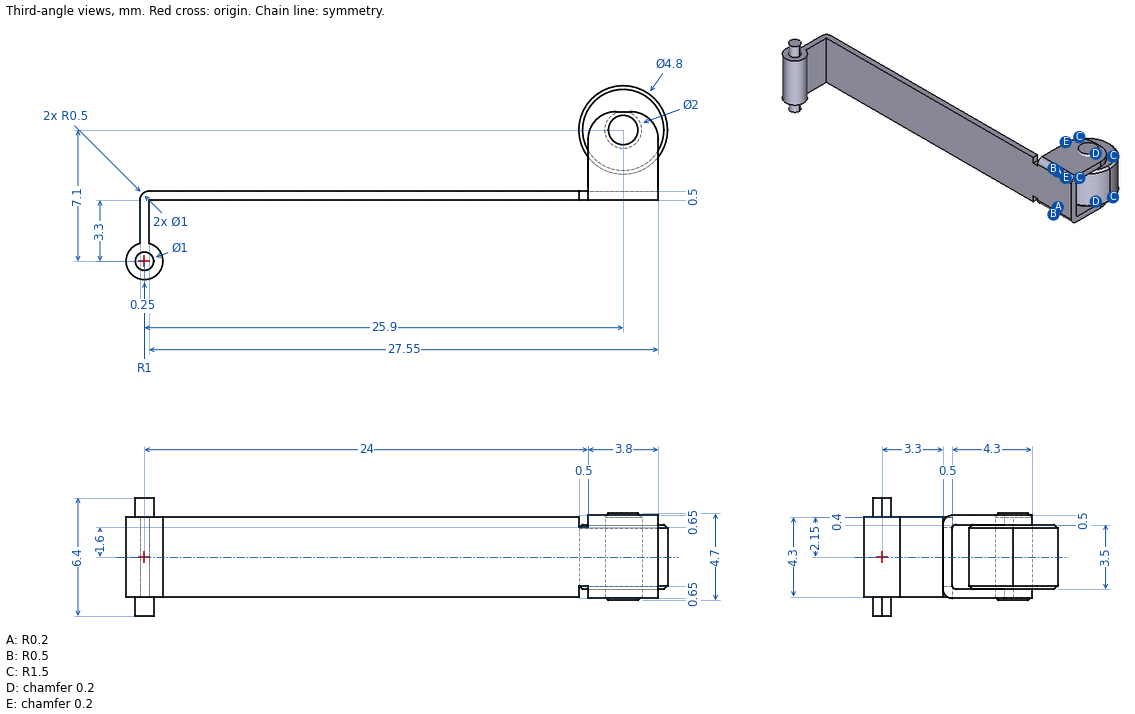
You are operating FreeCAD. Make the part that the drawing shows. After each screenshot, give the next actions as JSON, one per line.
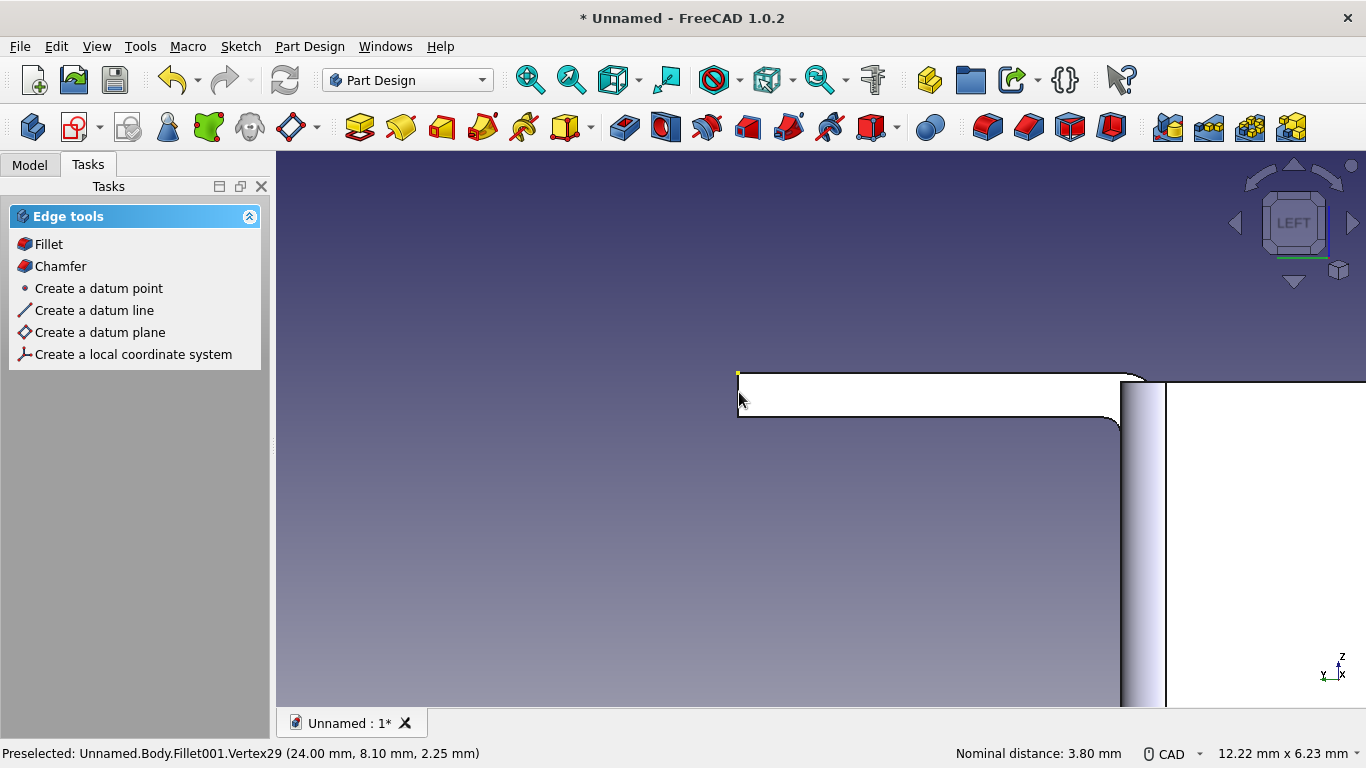
{"action": "left_click", "coordinate": [738, 394], "text": "ctrl"}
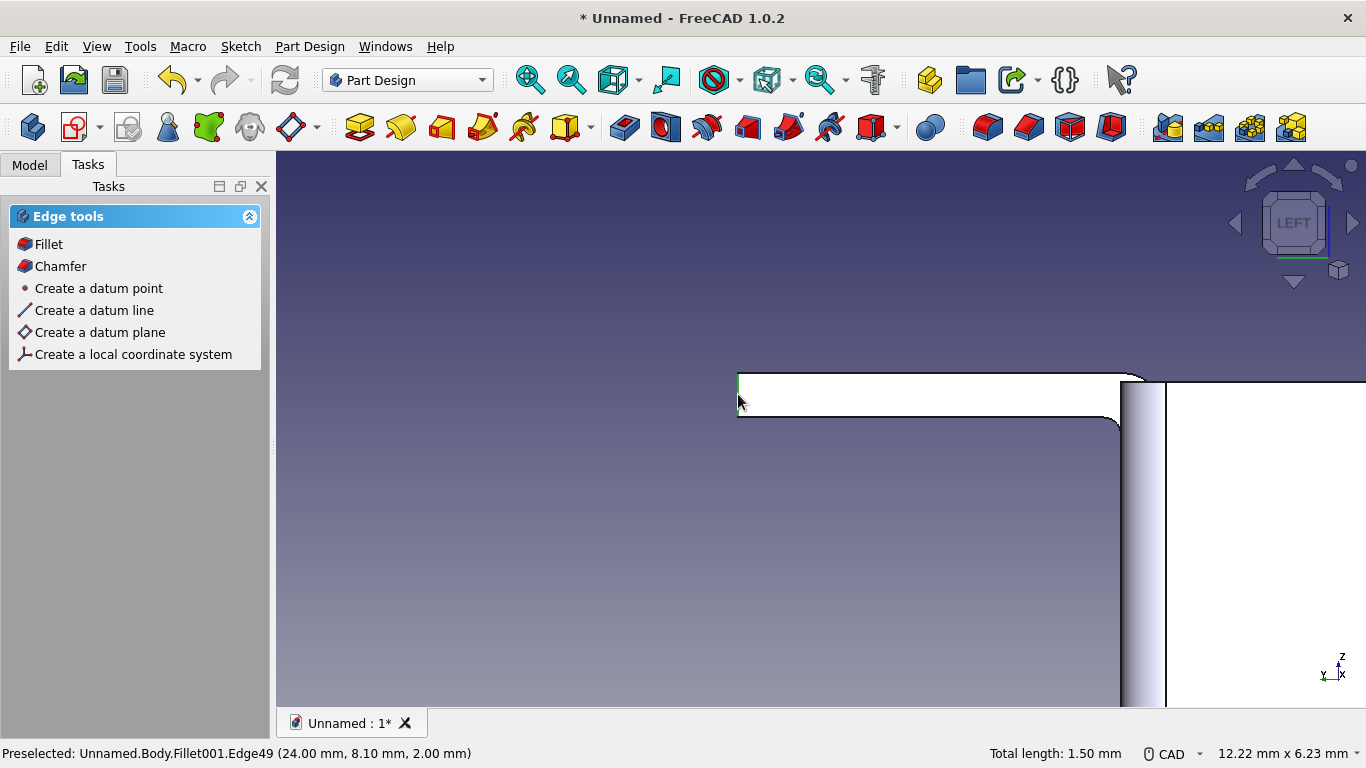
{"action": "key", "text": "v f"}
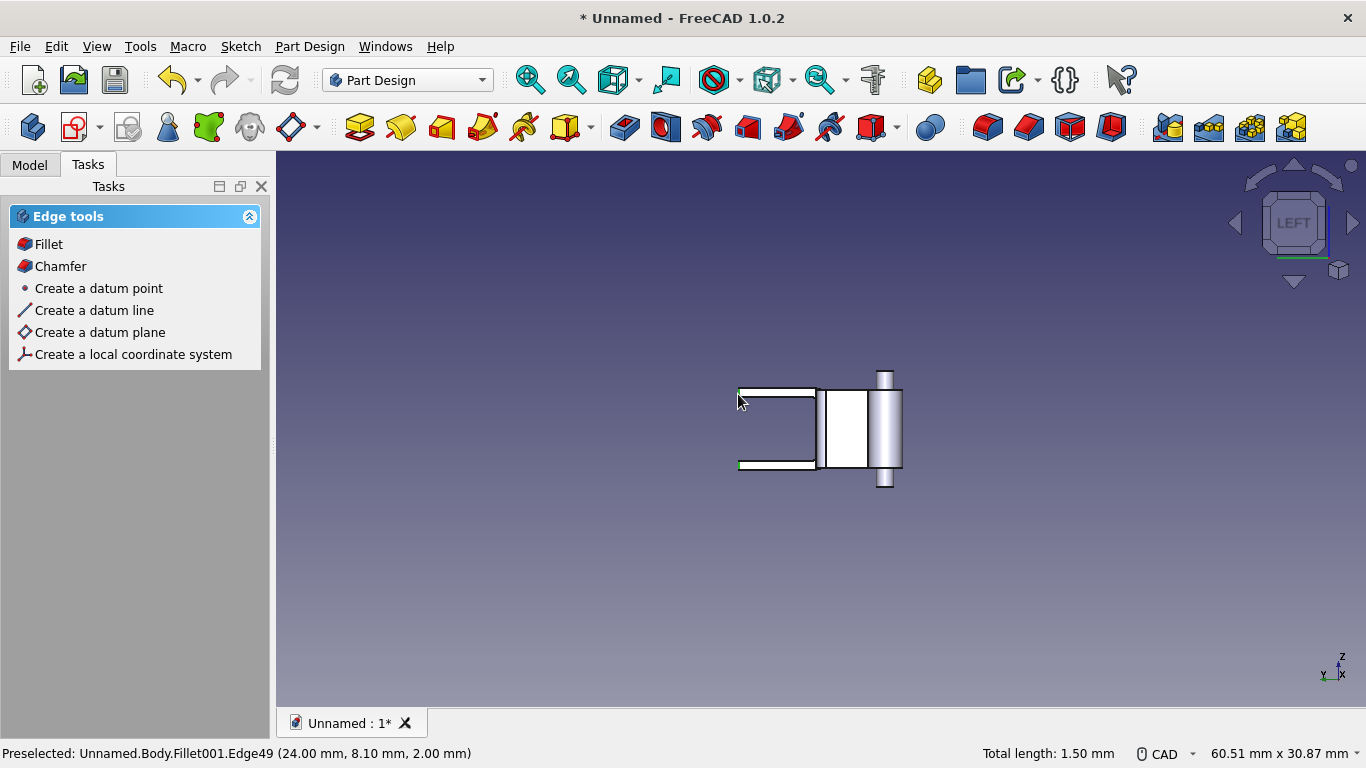
{"action": "key", "text": "v 3"}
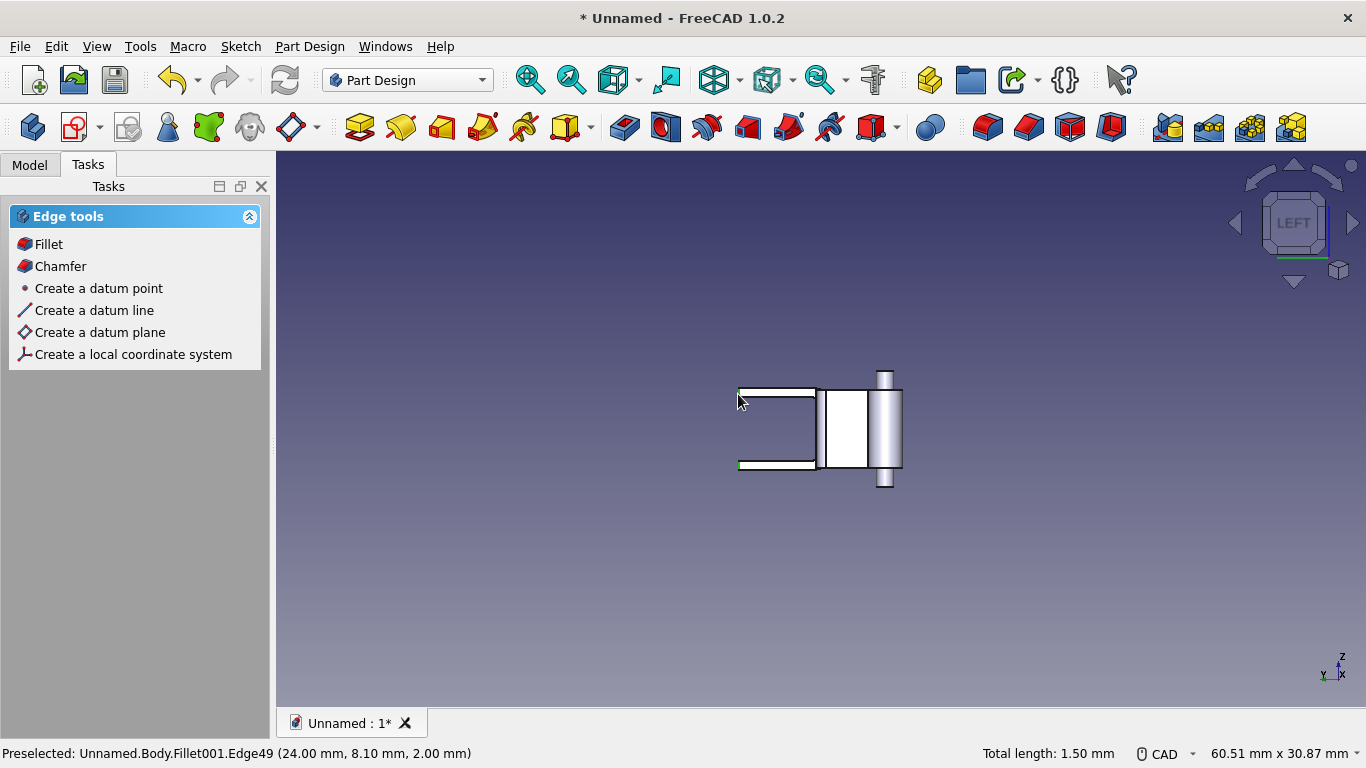
{"action": "key", "text": "0"}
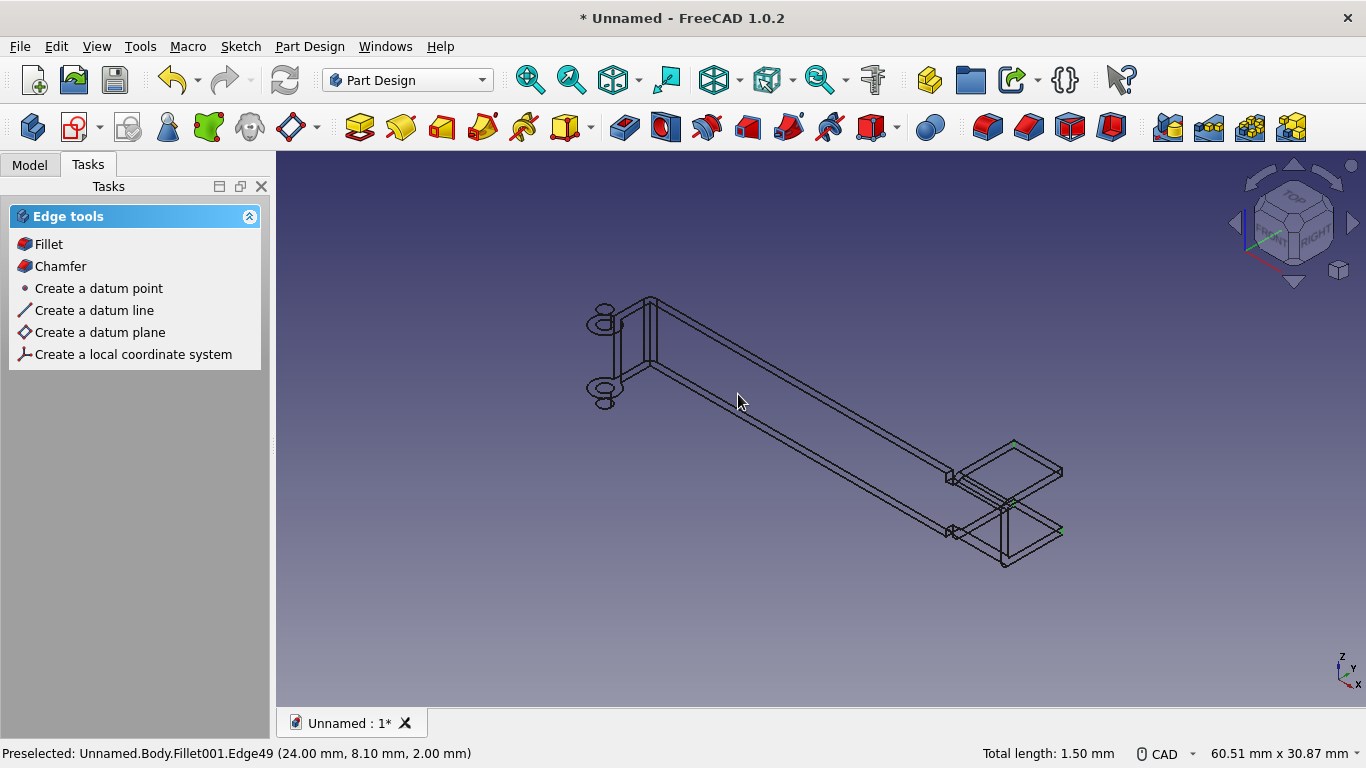
{"action": "scroll", "coordinate": [1062, 471], "scroll_direction": "up", "scroll_amount": 8}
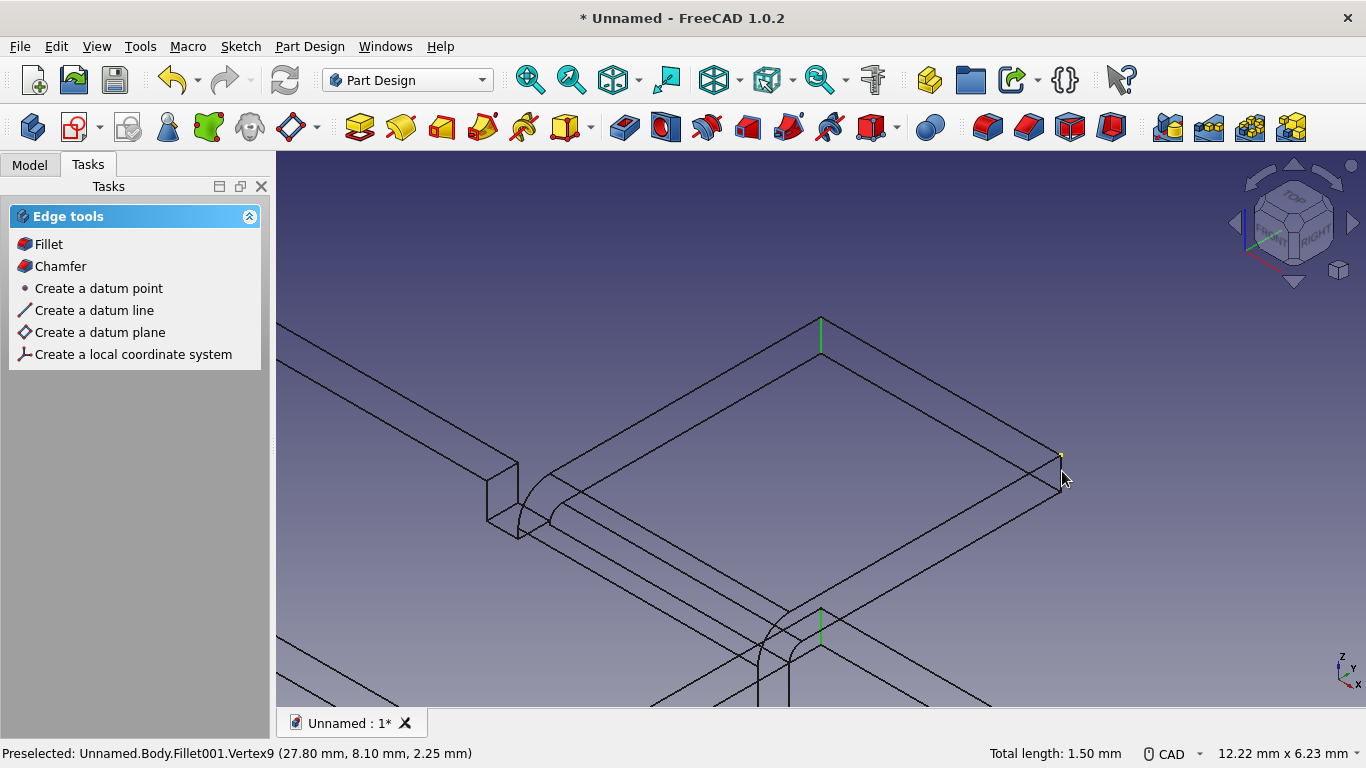
{"action": "left_click", "coordinate": [1061, 473], "text": "ctrl"}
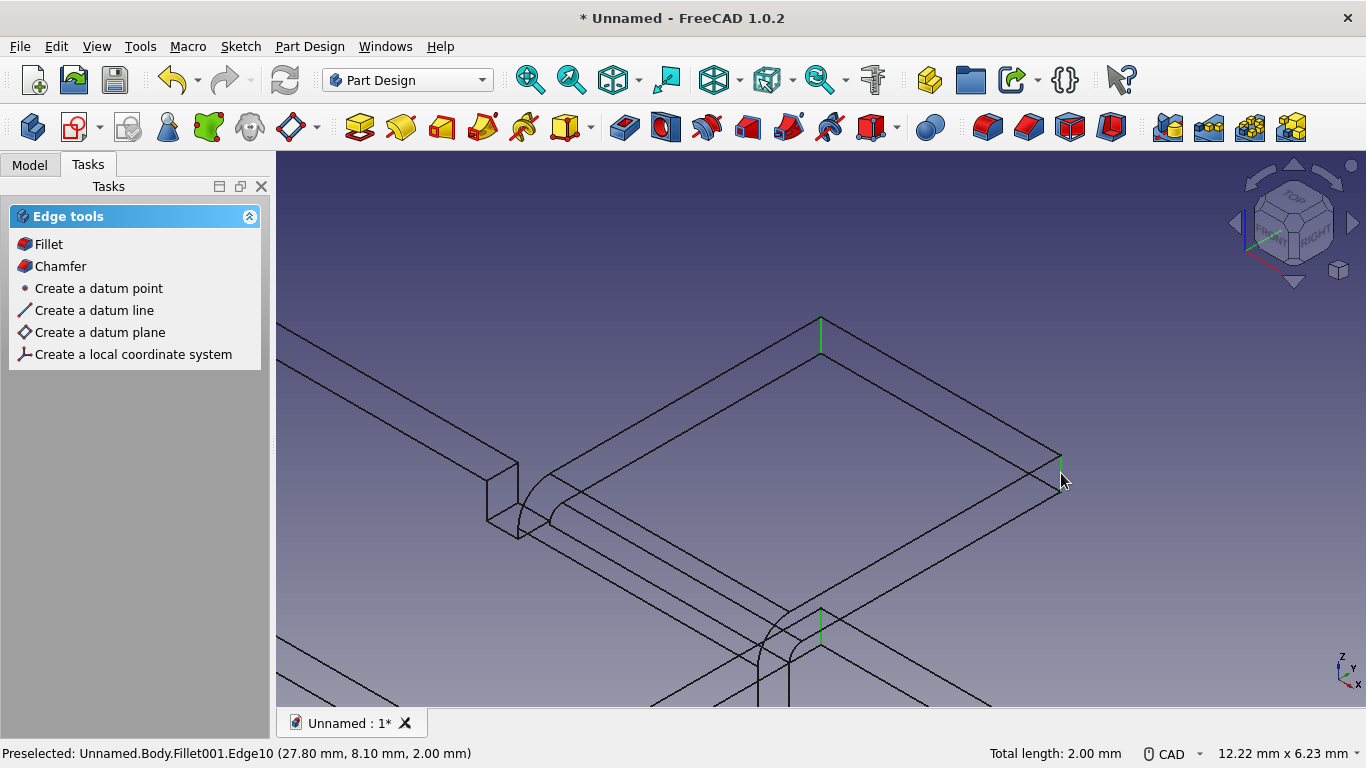
{"action": "key", "text": "v 1"}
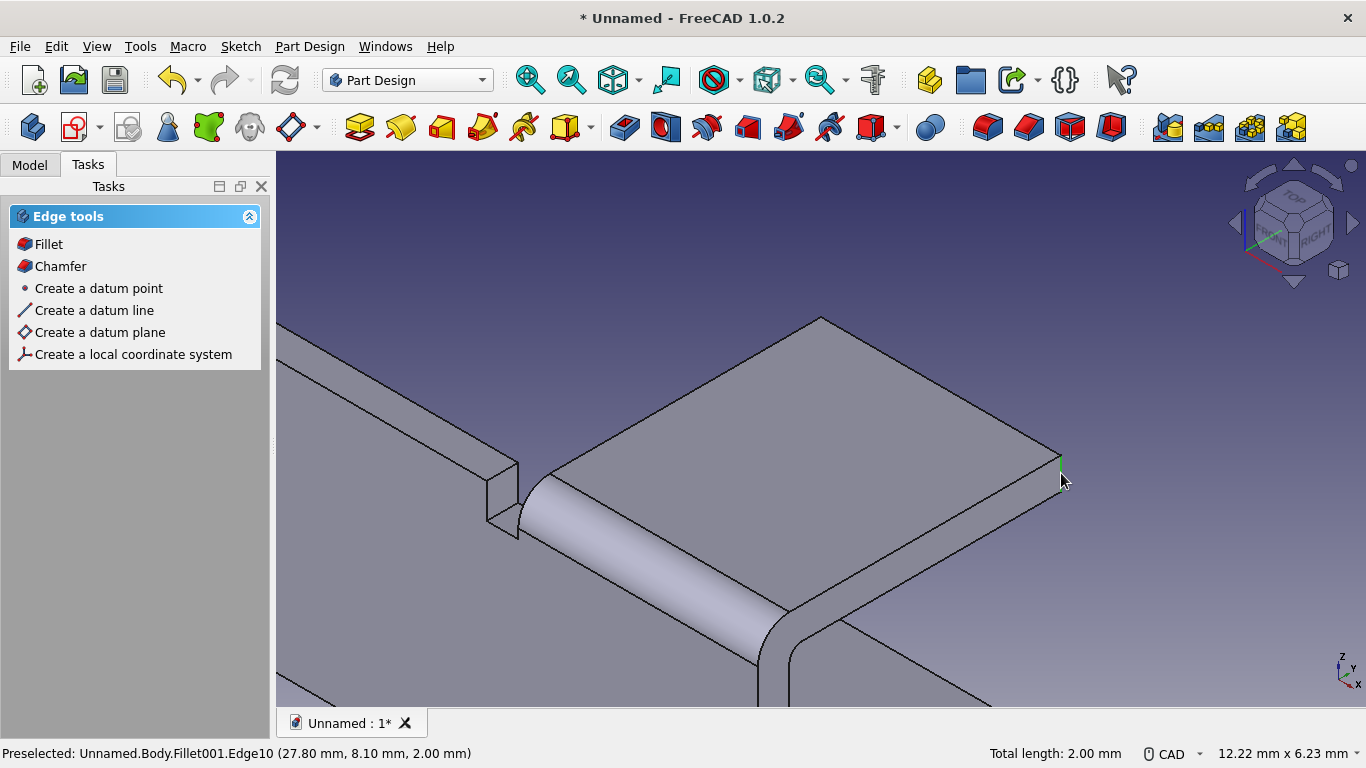
{"action": "left_click", "coordinate": [988, 128]}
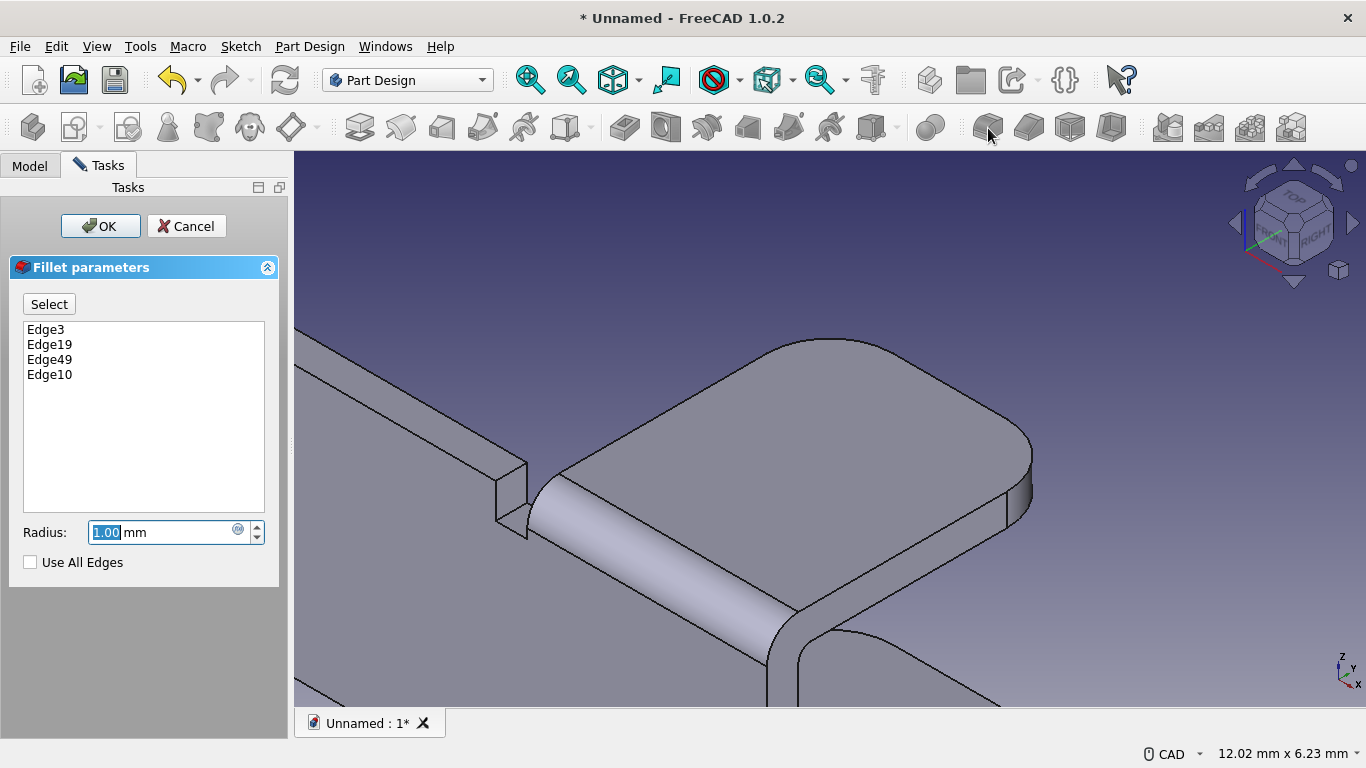
{"action": "type", "text": "1.5"}
{"action": "key", "text": "Tab"}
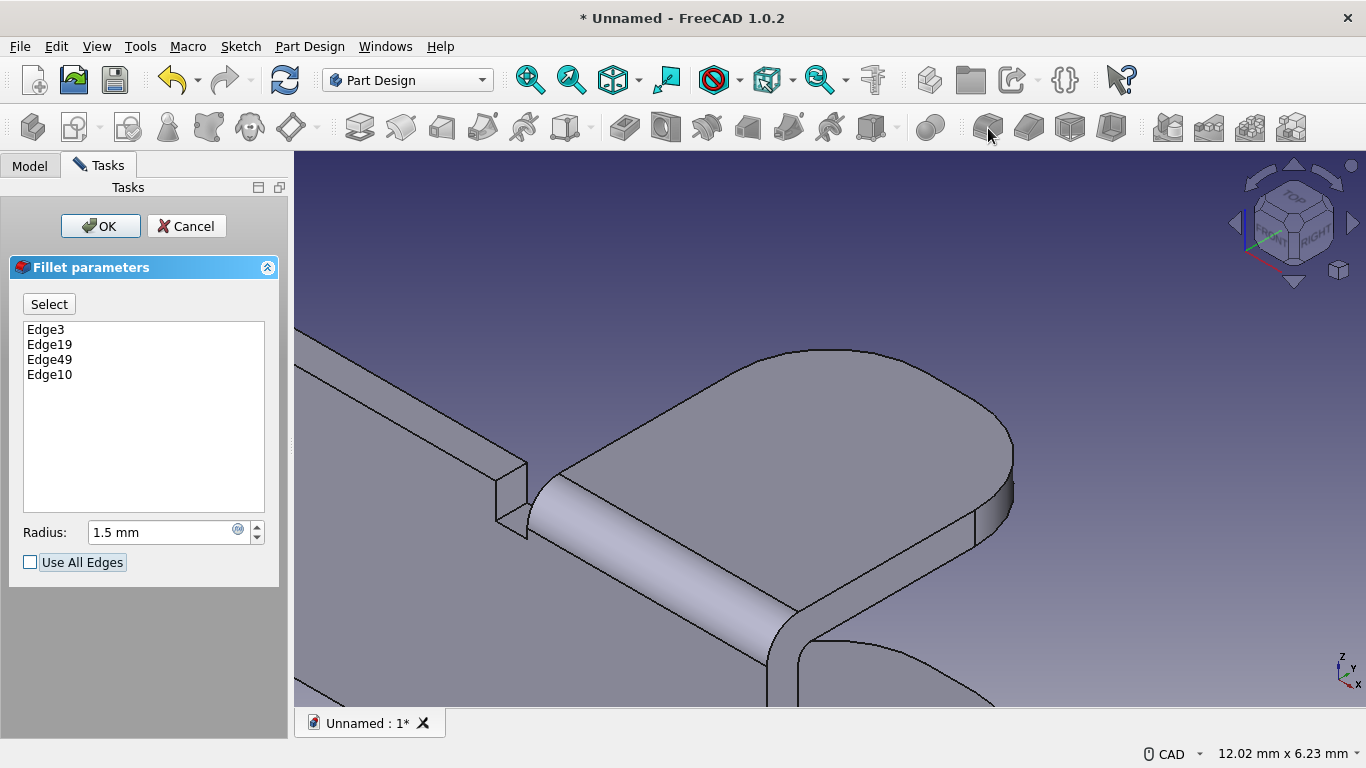
{"action": "left_click", "coordinate": [101, 226]}